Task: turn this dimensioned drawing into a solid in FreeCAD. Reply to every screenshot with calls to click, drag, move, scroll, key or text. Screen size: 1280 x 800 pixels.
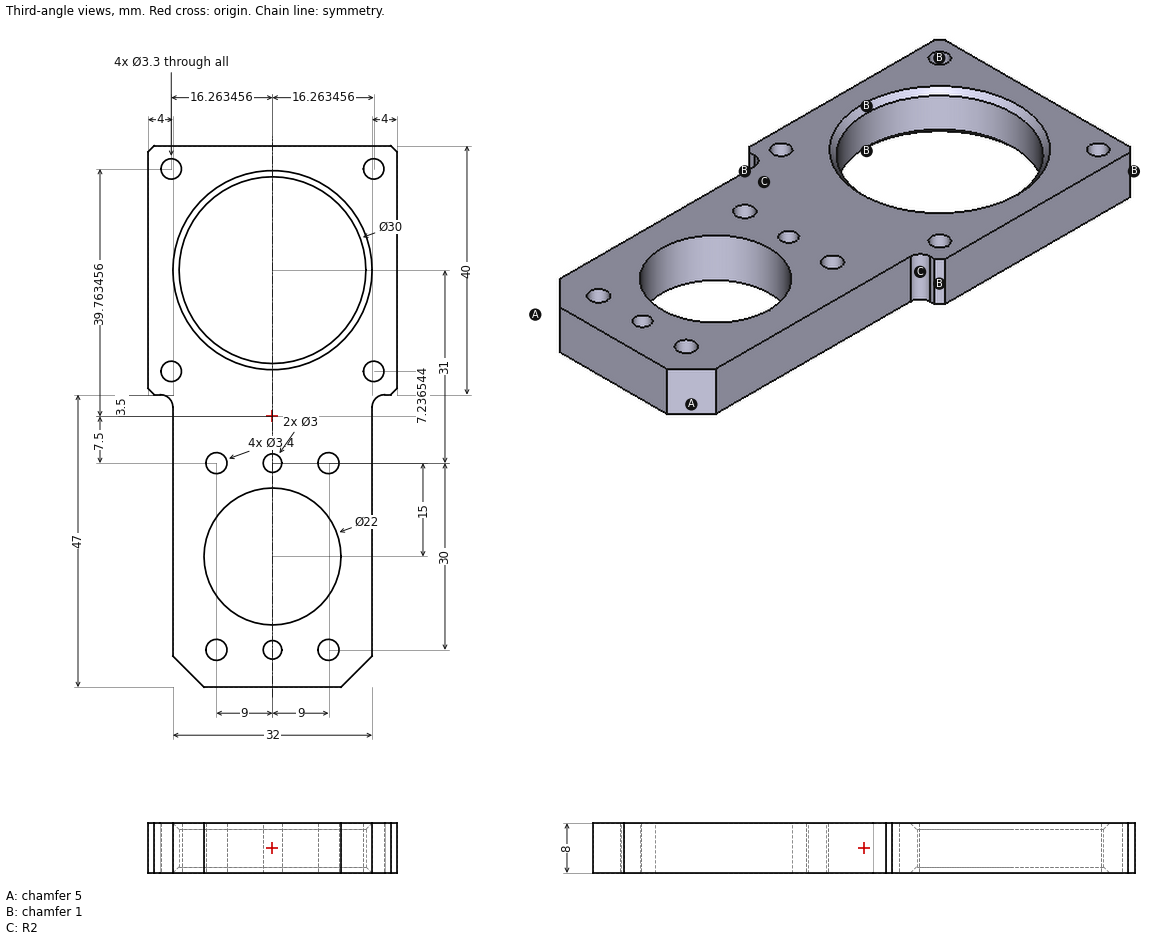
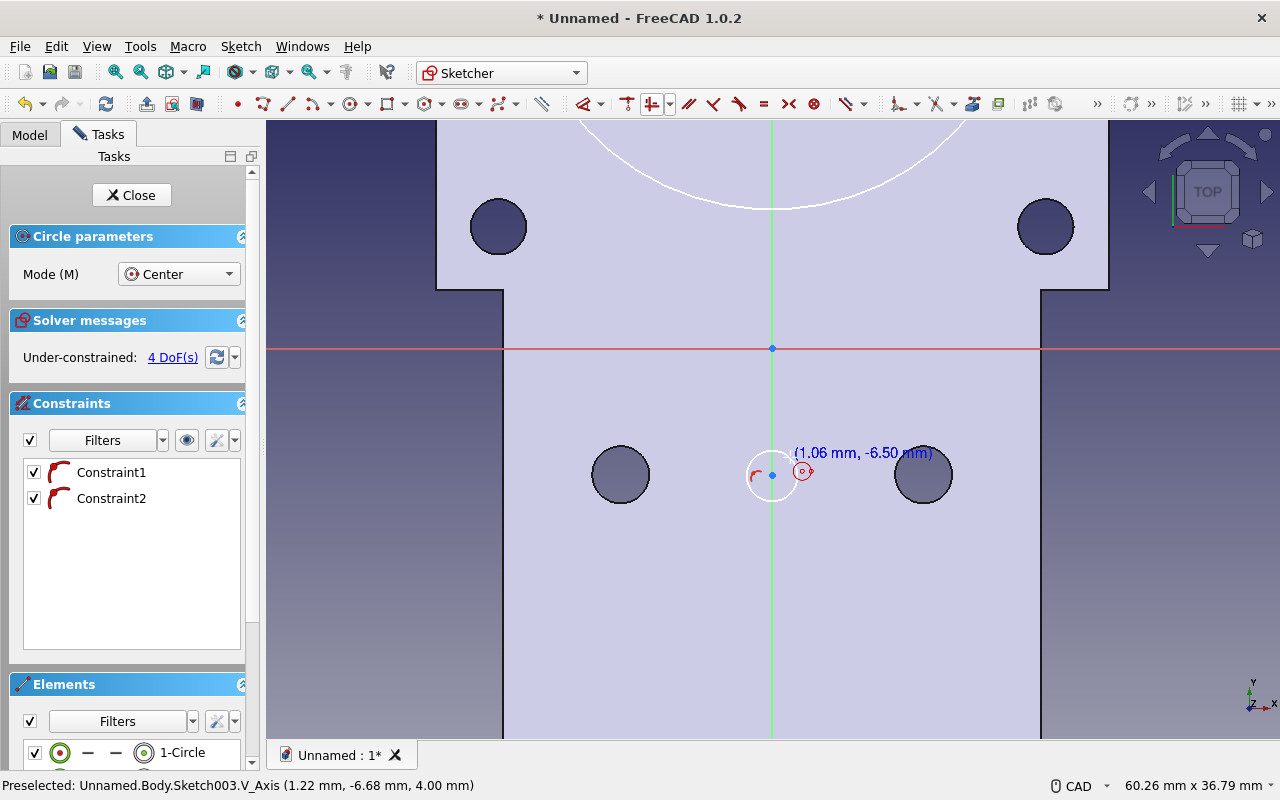
scroll(675, 463, down, 6)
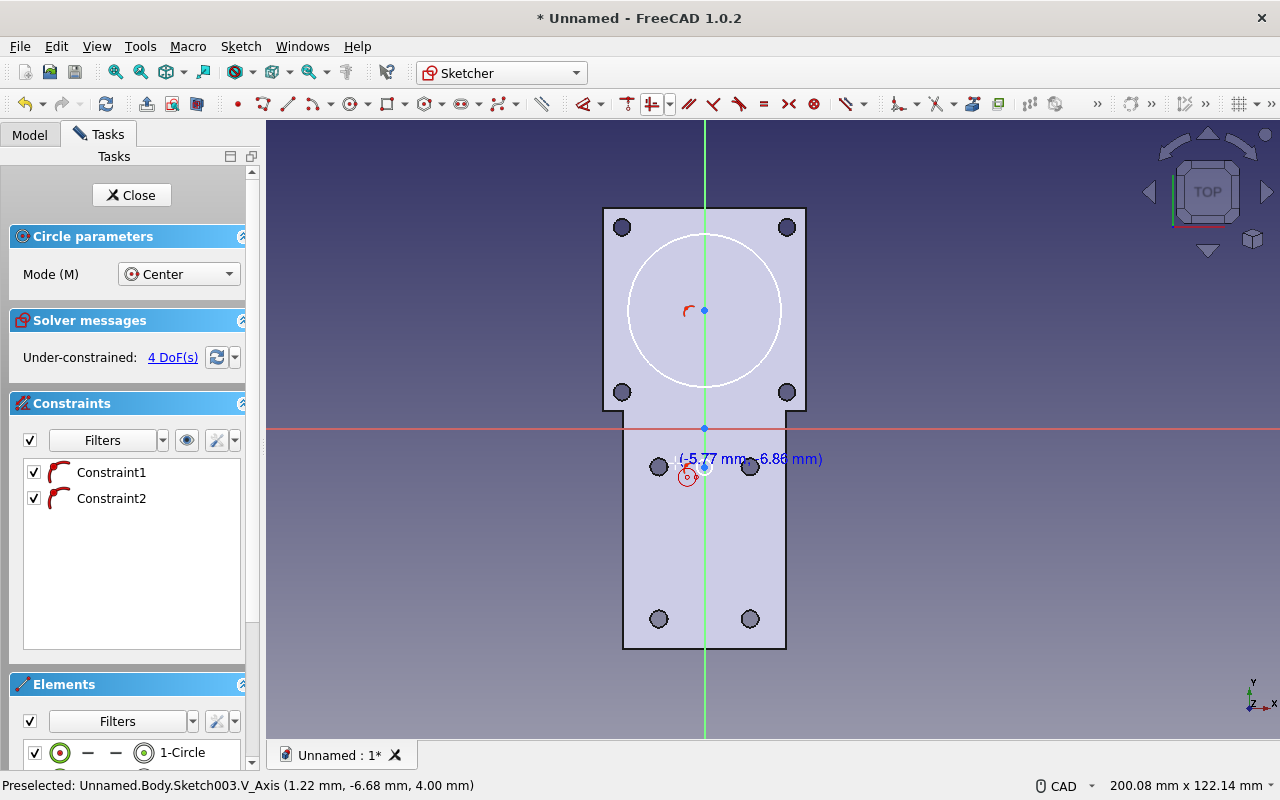
scroll(705, 619, up, 6)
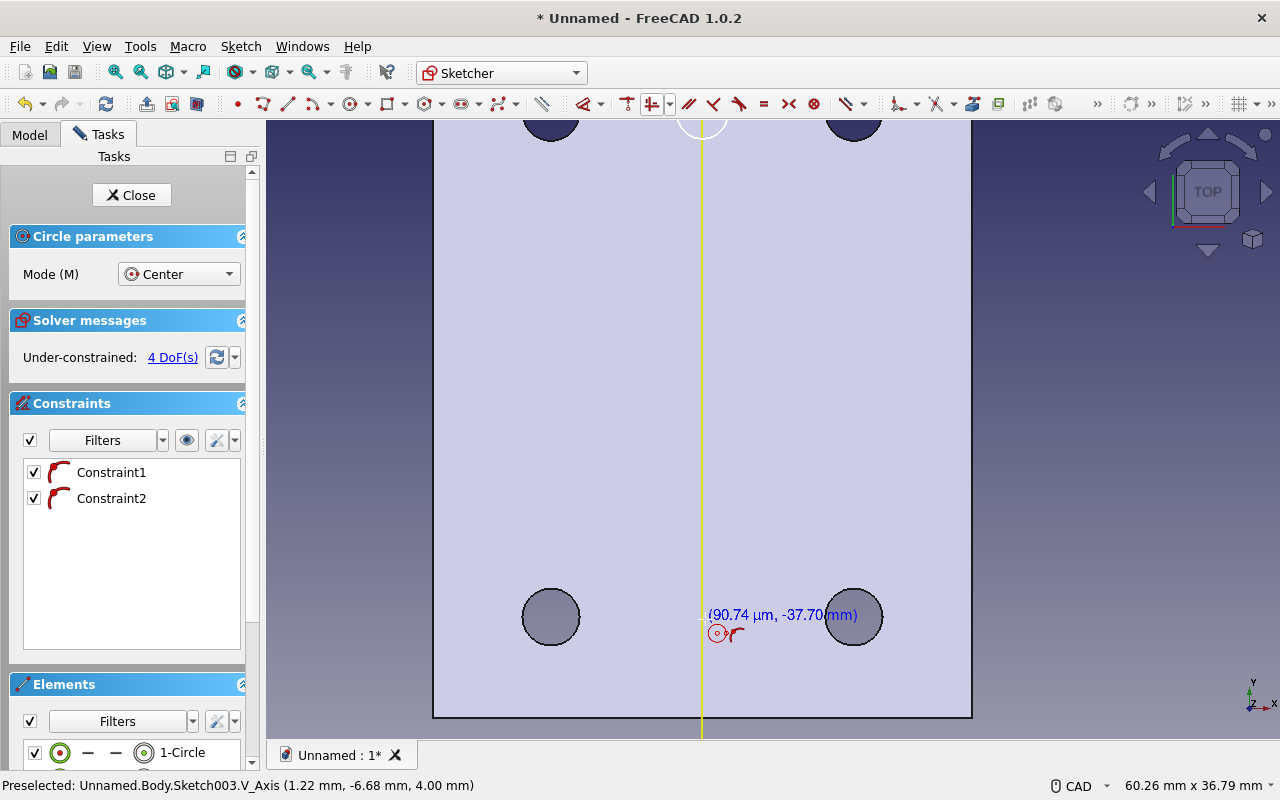
click(702, 617)
click(720, 599)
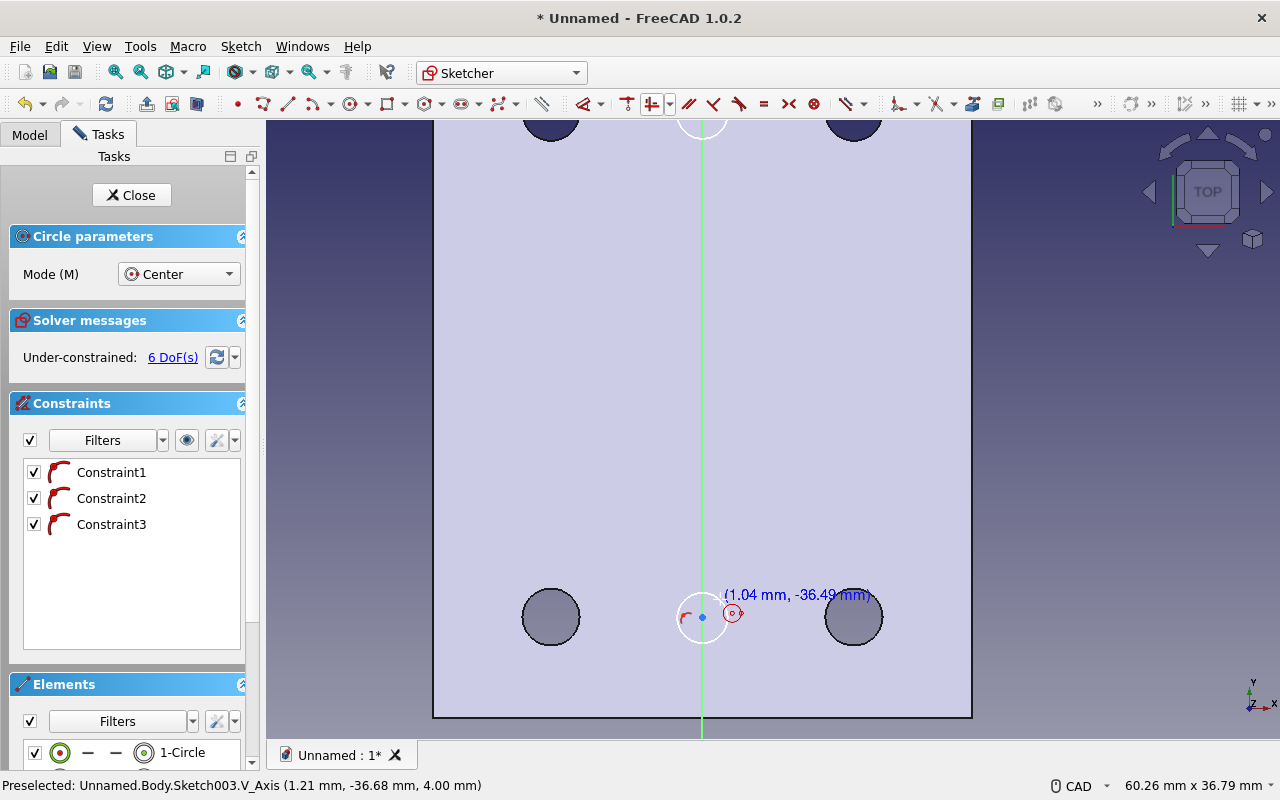
click(702, 365)
click(833, 234)
key(Escape)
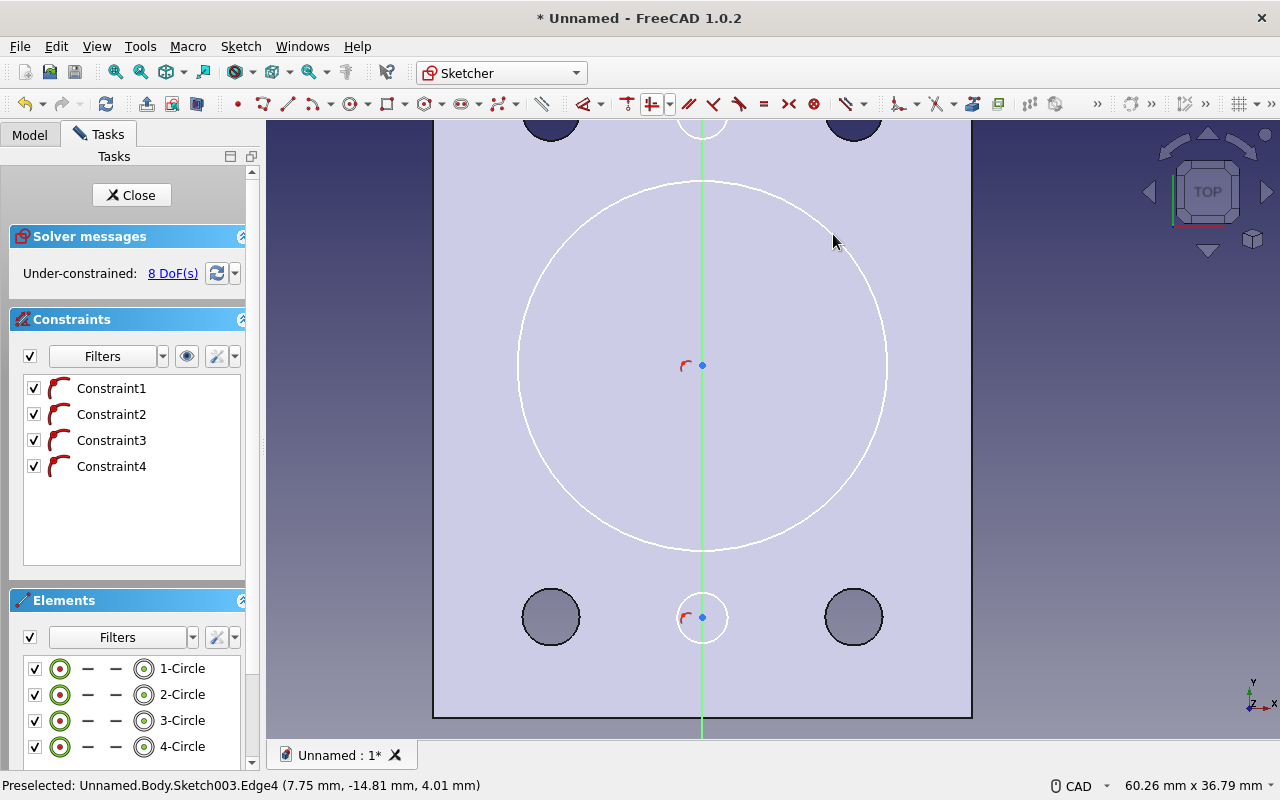
scroll(705, 619, down, 6)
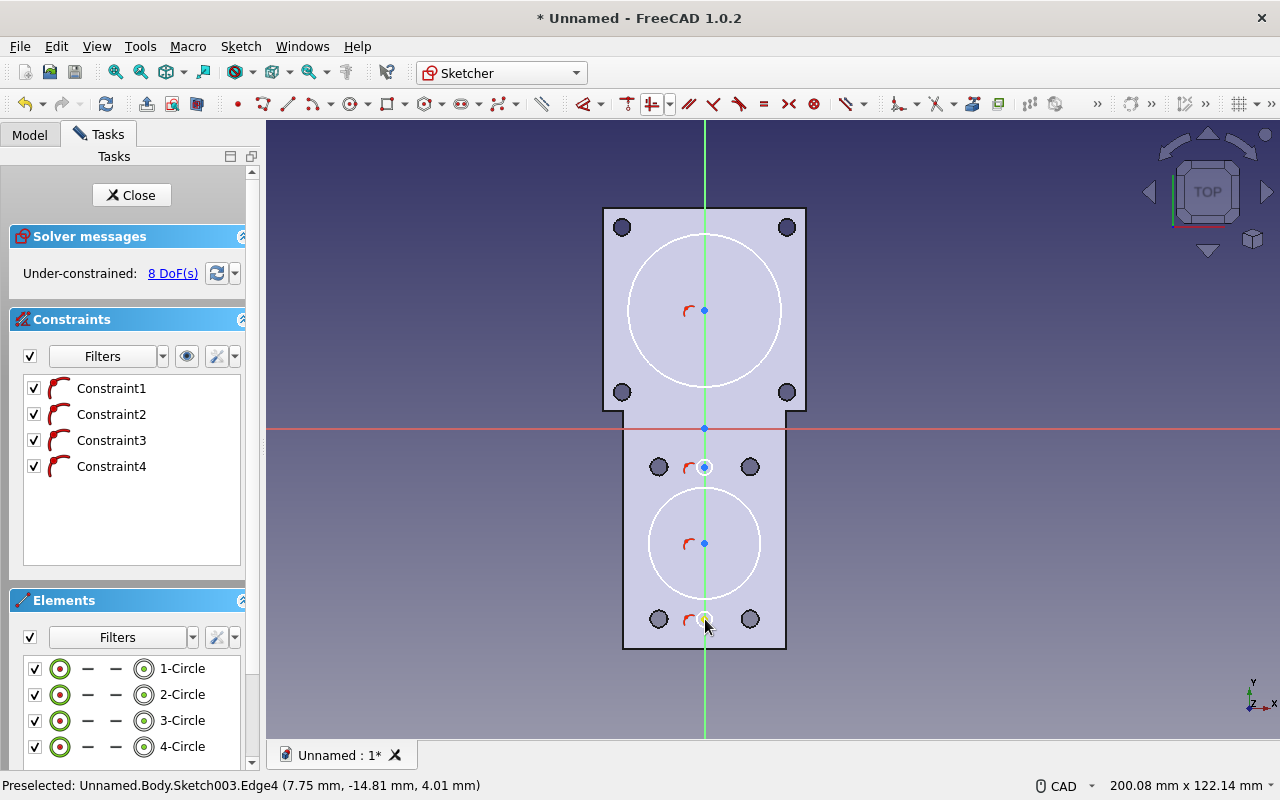
scroll(710, 462, up, 5)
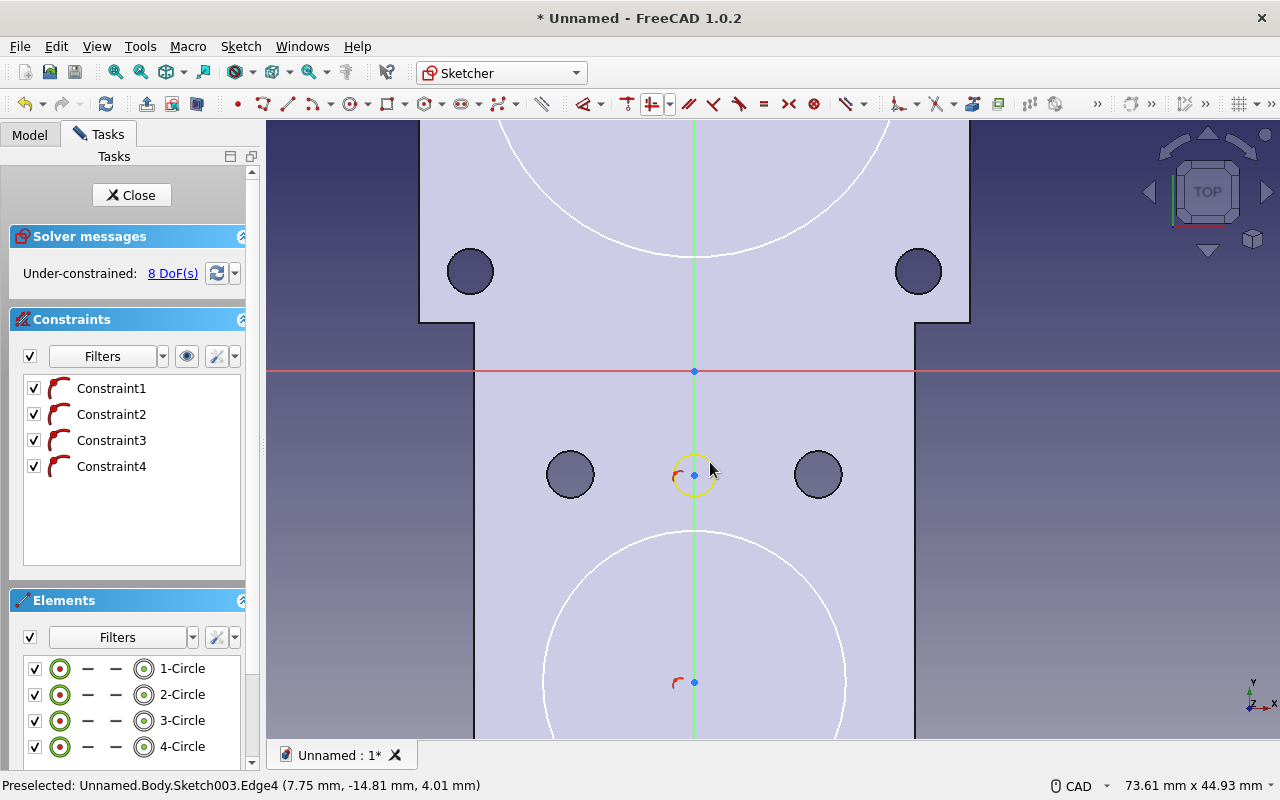
click(709, 461)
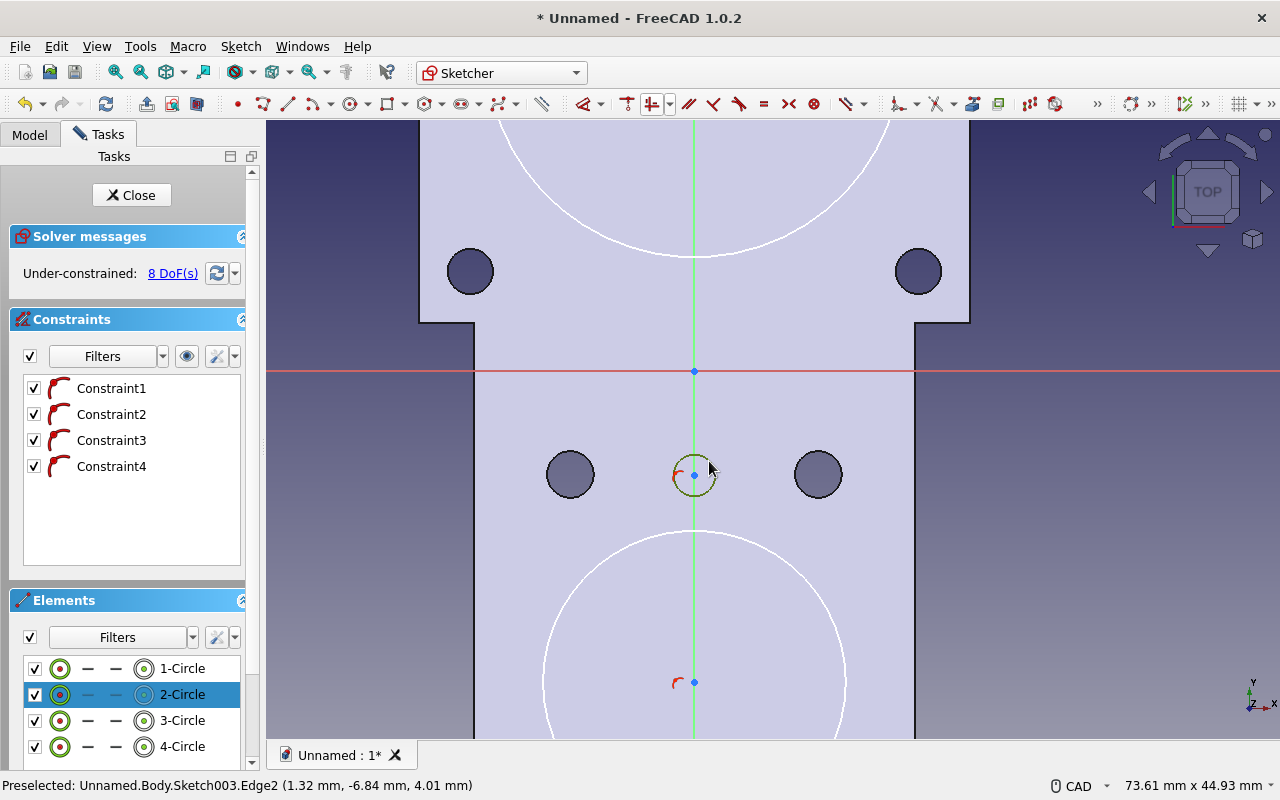
scroll(710, 461, down, 5)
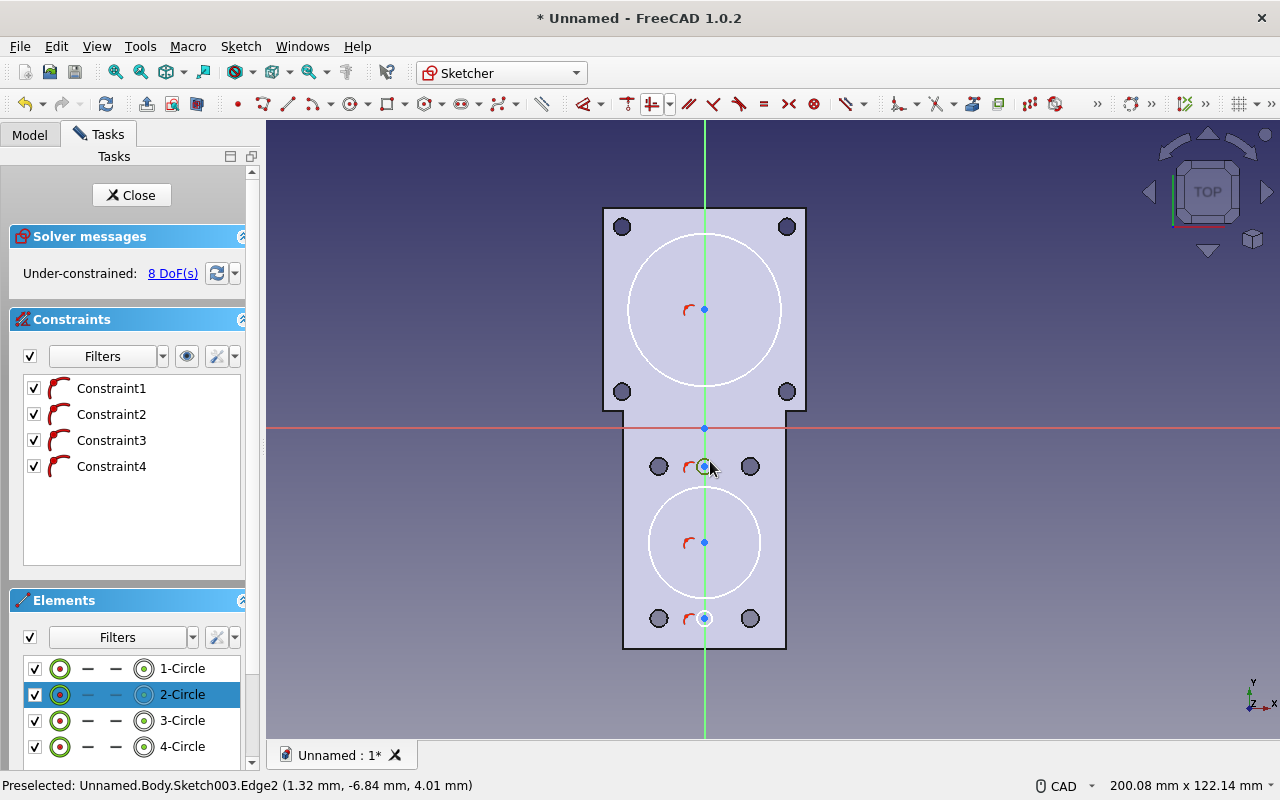
scroll(710, 613, up, 5)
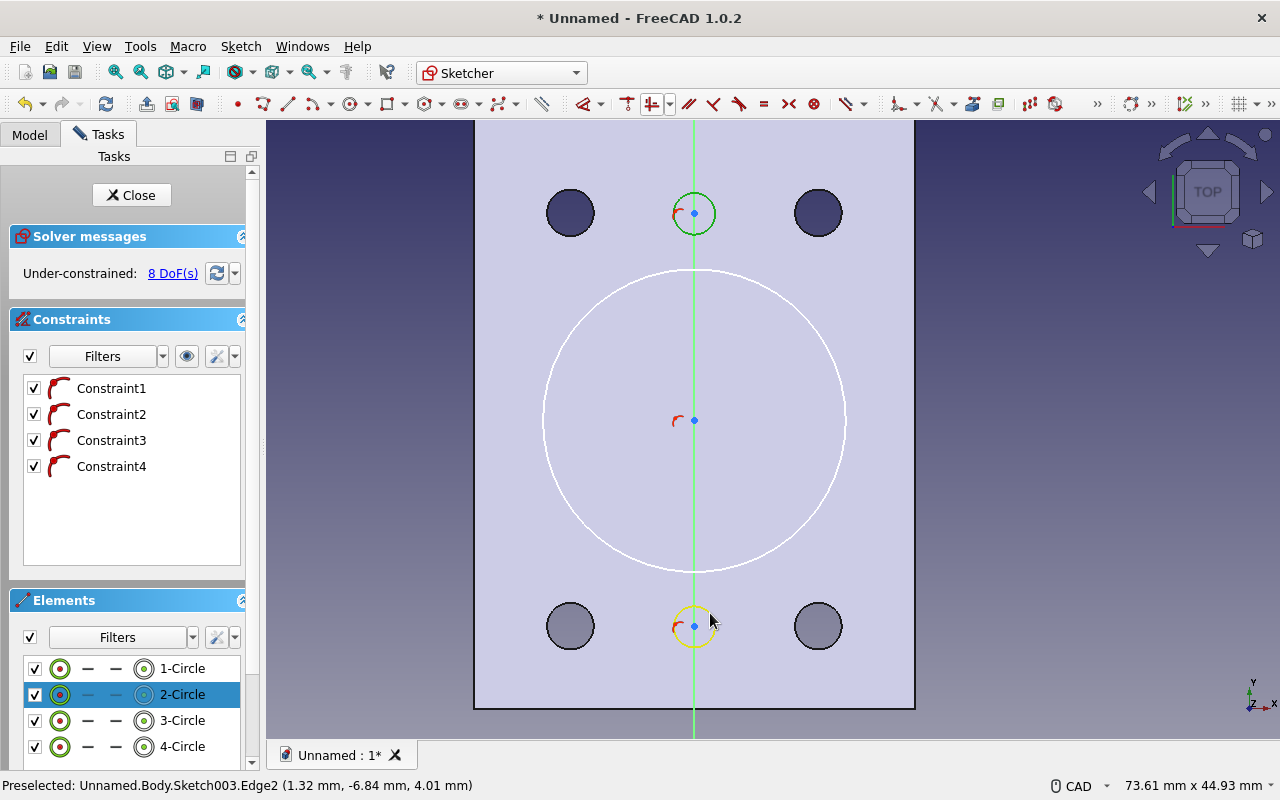
click(709, 612)